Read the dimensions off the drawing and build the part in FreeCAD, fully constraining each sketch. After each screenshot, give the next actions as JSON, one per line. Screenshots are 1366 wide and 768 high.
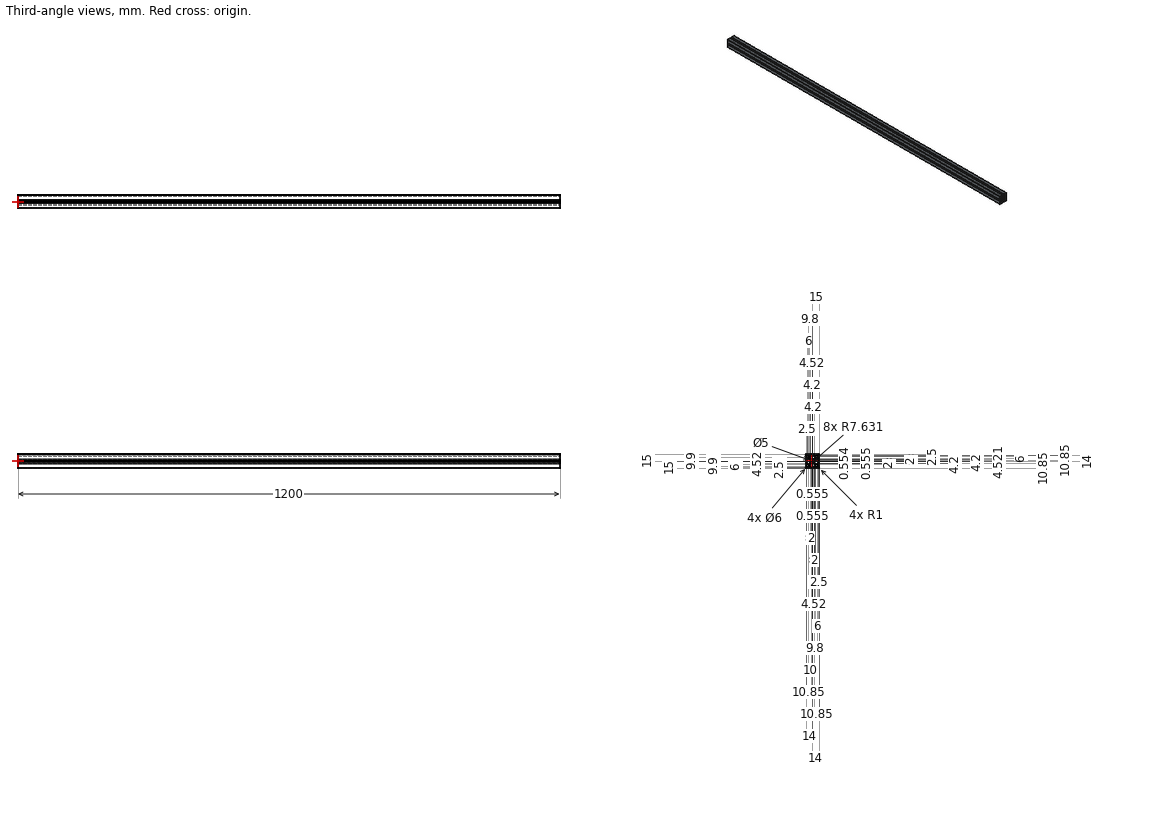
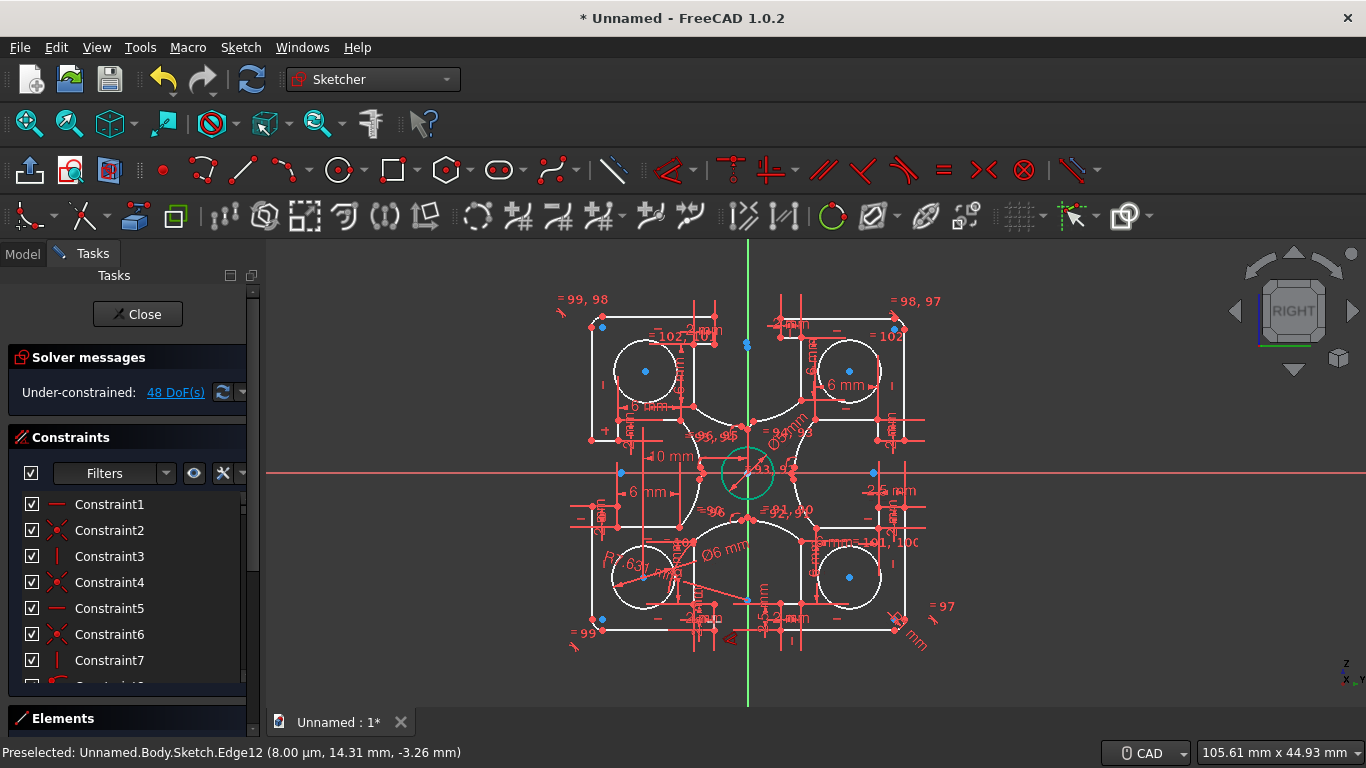
{"action": "scroll", "coordinate": [886, 441], "scroll_direction": "up", "scroll_amount": 3}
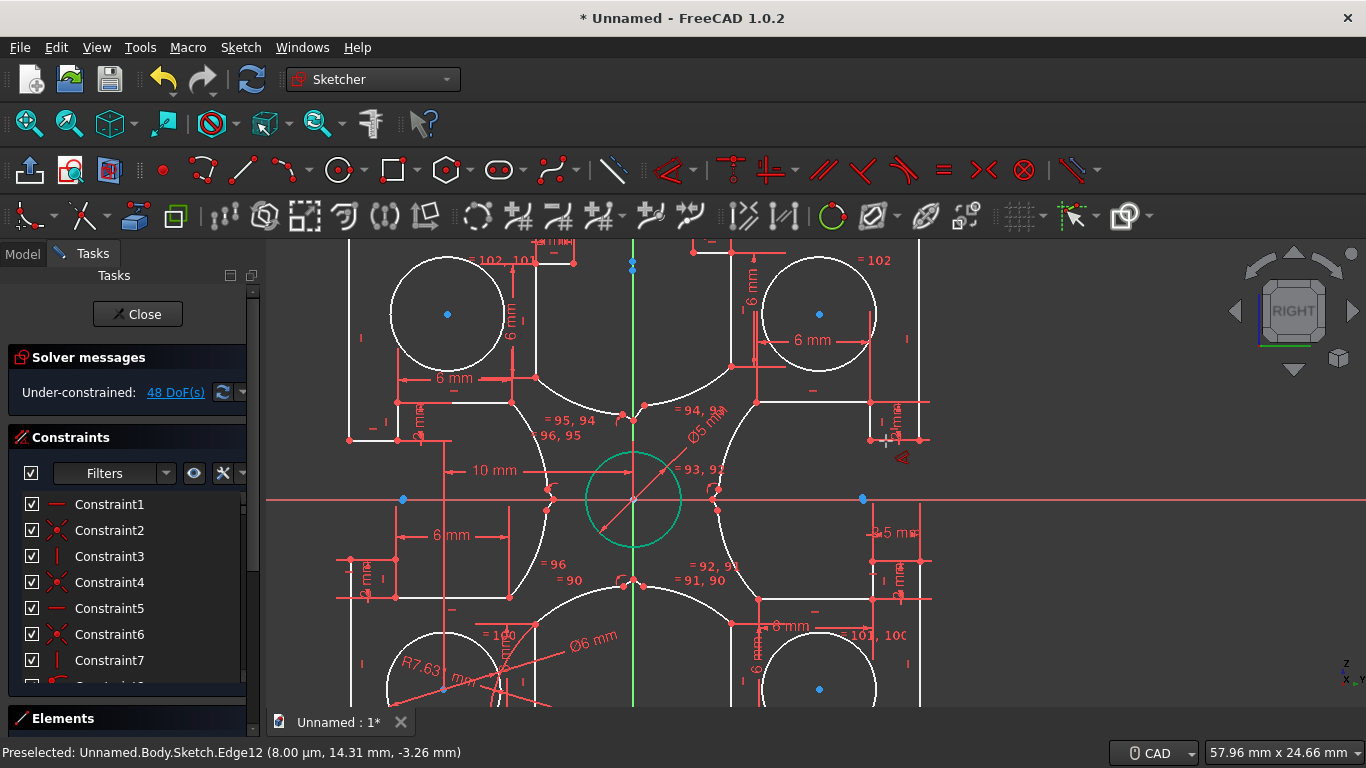
{"action": "left_click", "coordinate": [885, 440]}
{"action": "left_click", "coordinate": [895, 474]}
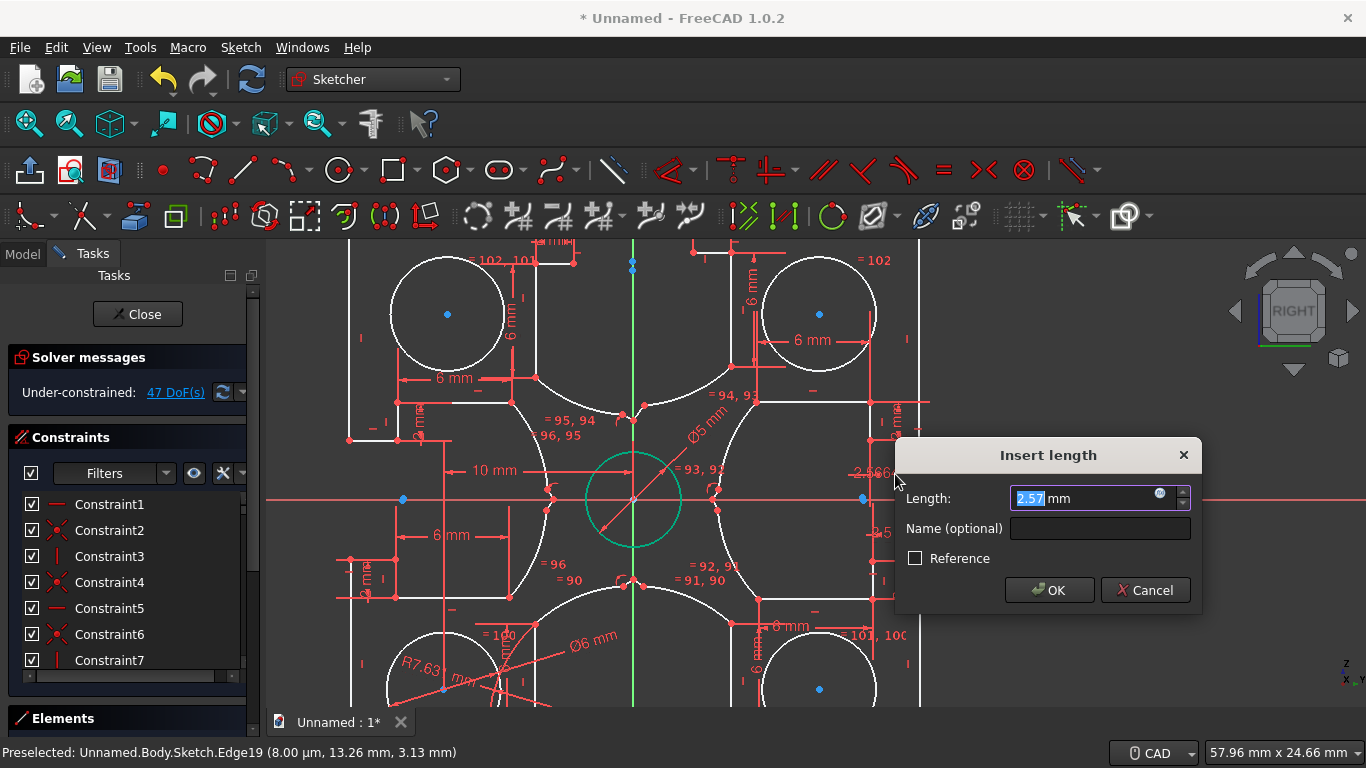
{"action": "type", "text": "2.5"}
{"action": "key", "text": "Return"}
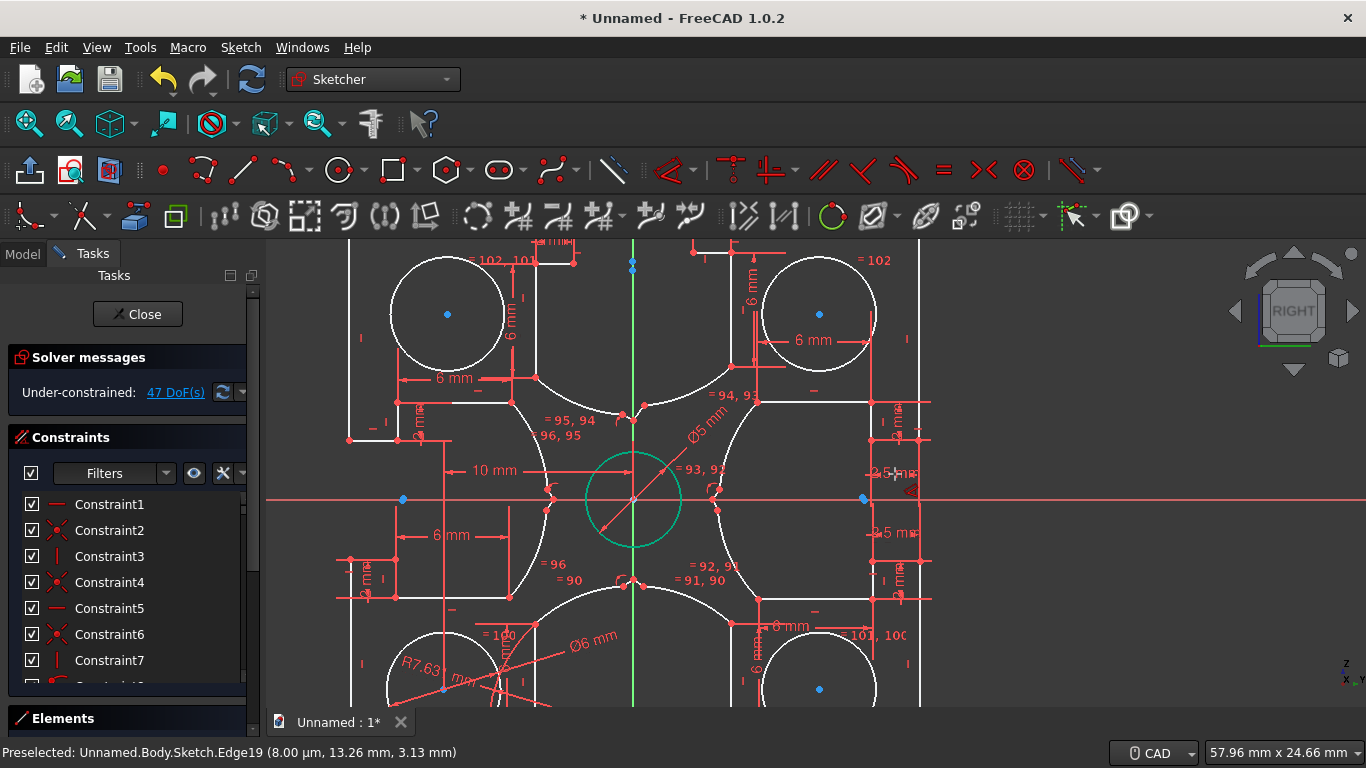
{"action": "scroll", "coordinate": [886, 441], "scroll_direction": "down", "scroll_amount": 3}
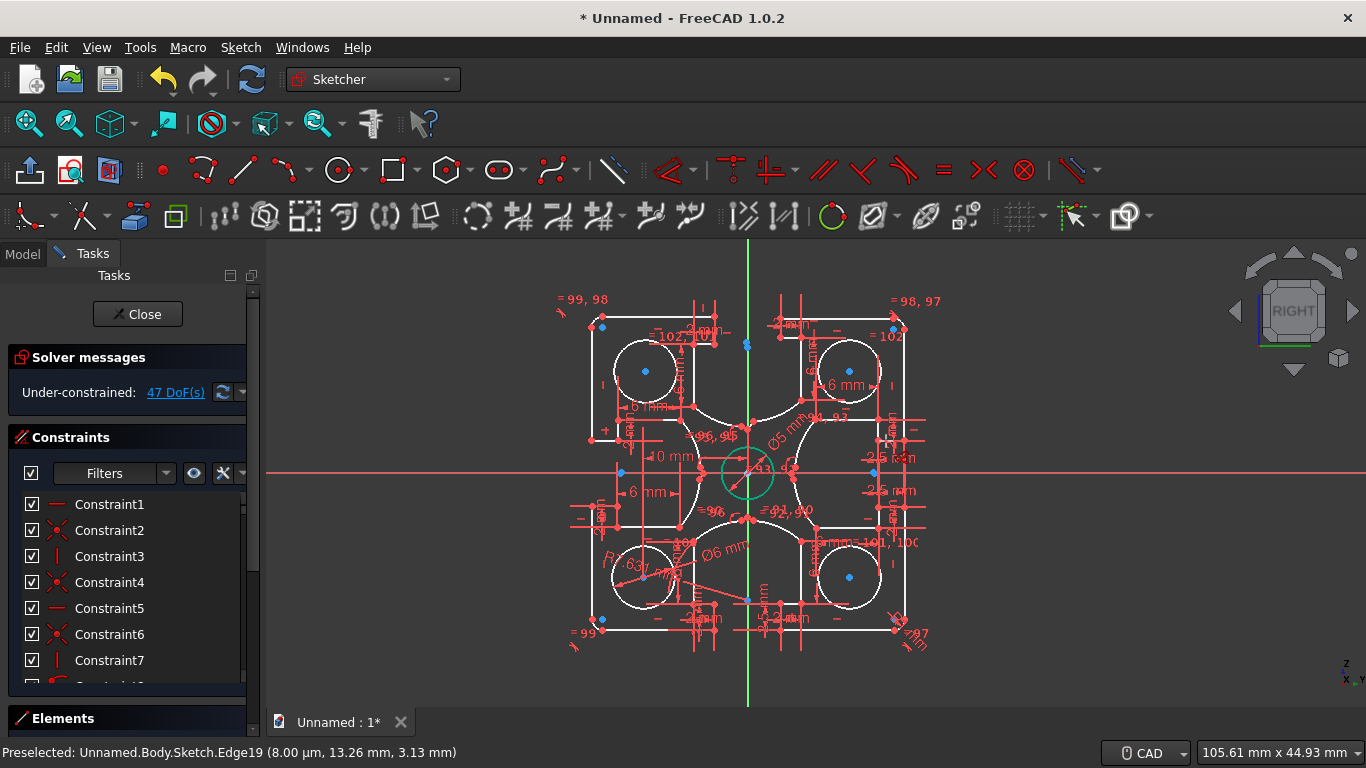
{"action": "scroll", "coordinate": [781, 325], "scroll_direction": "up", "scroll_amount": 5}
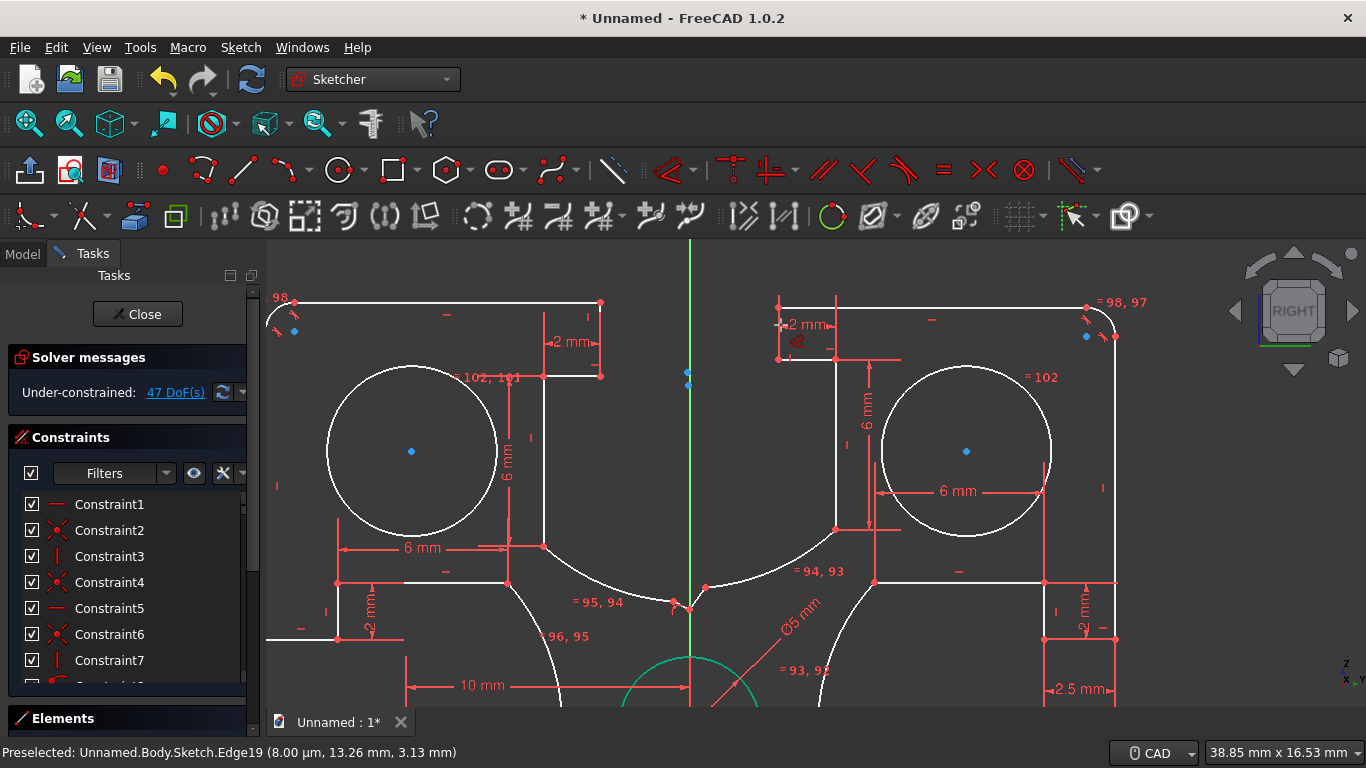
{"action": "left_click", "coordinate": [779, 323]}
{"action": "left_click", "coordinate": [813, 322]}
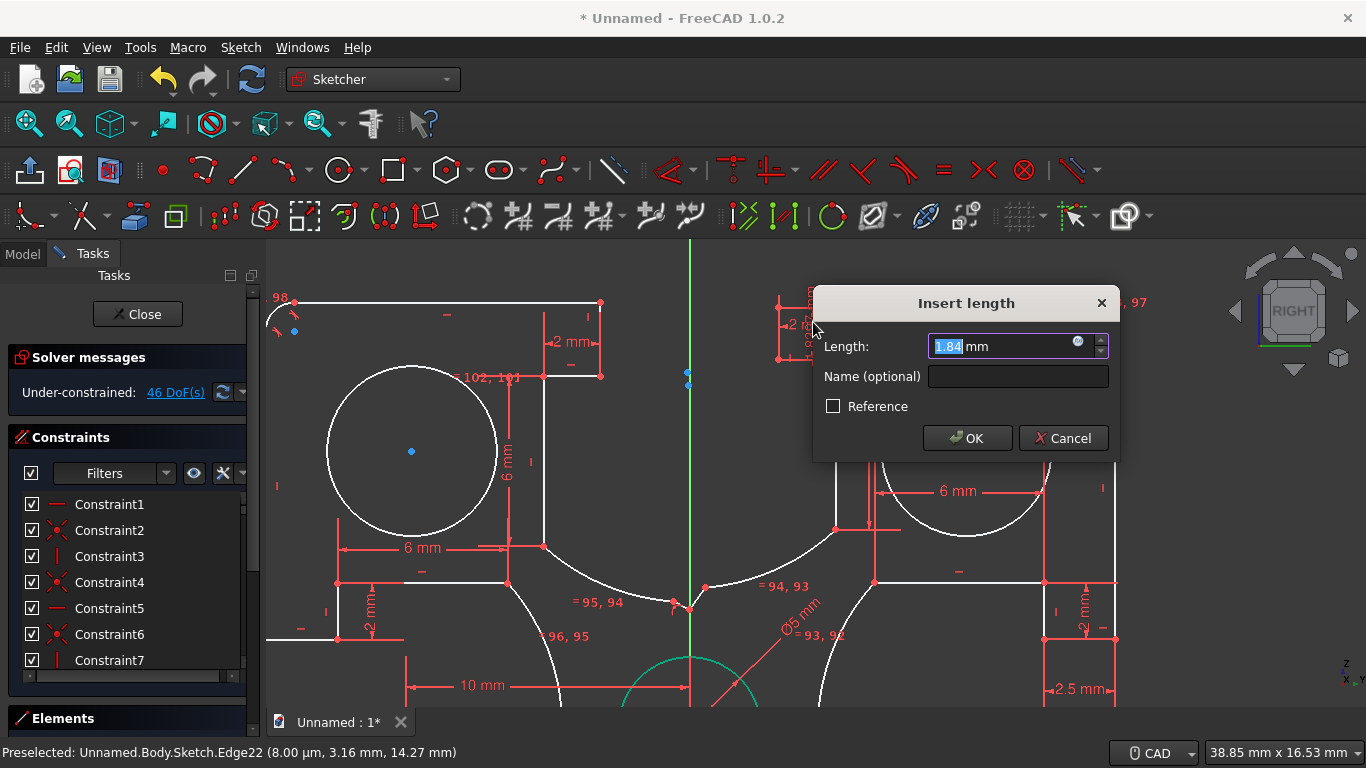
{"action": "type", "text": "2.5"}
{"action": "key", "text": "Return"}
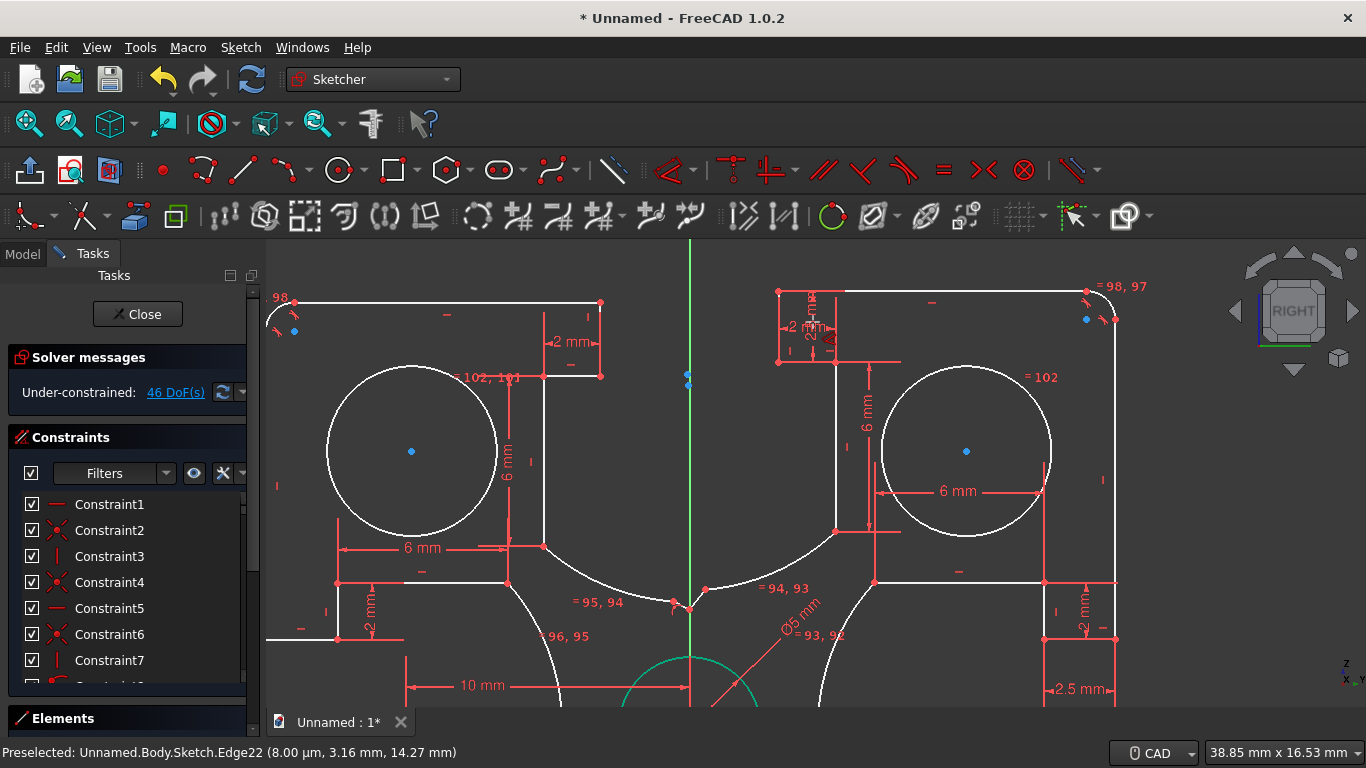
{"action": "left_click", "coordinate": [600, 354]}
{"action": "left_click", "coordinate": [634, 314]}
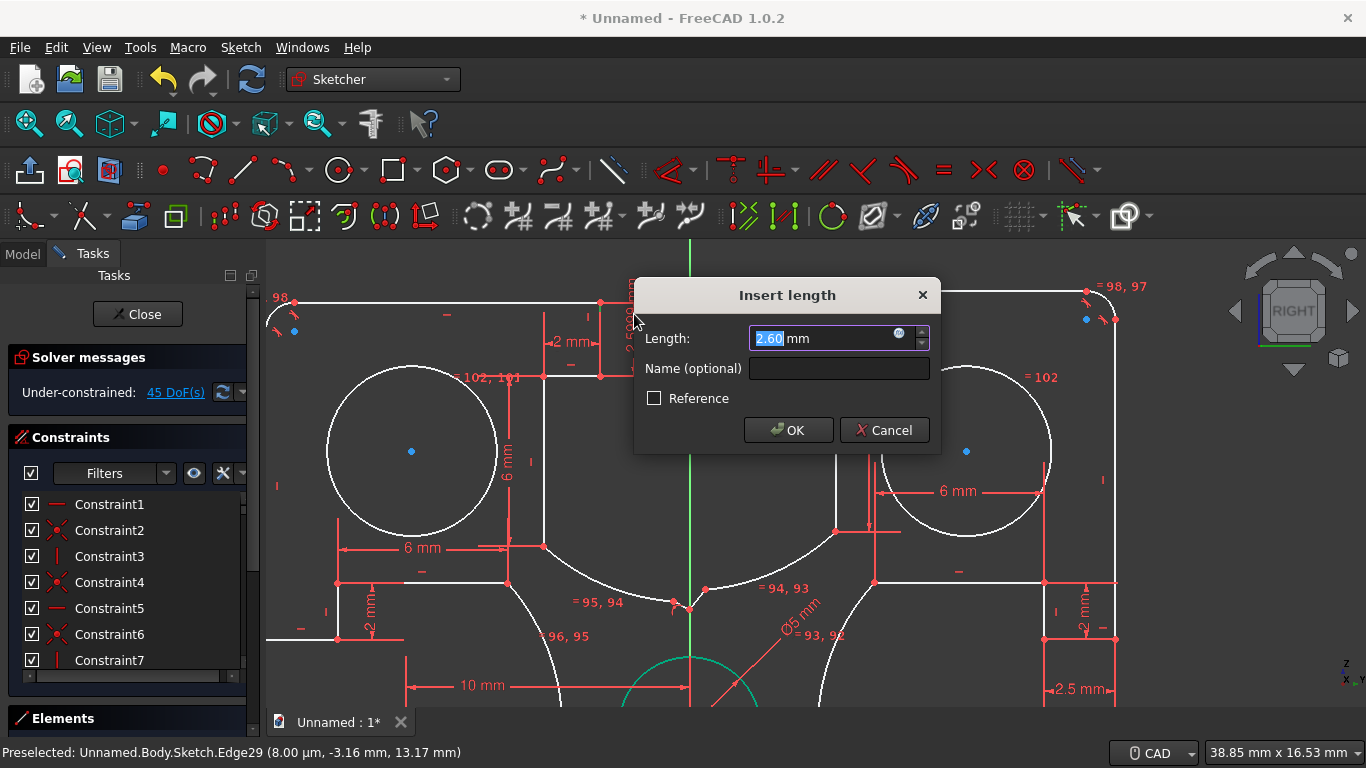
{"action": "type", "text": "2.5"}
{"action": "key", "text": "Return"}